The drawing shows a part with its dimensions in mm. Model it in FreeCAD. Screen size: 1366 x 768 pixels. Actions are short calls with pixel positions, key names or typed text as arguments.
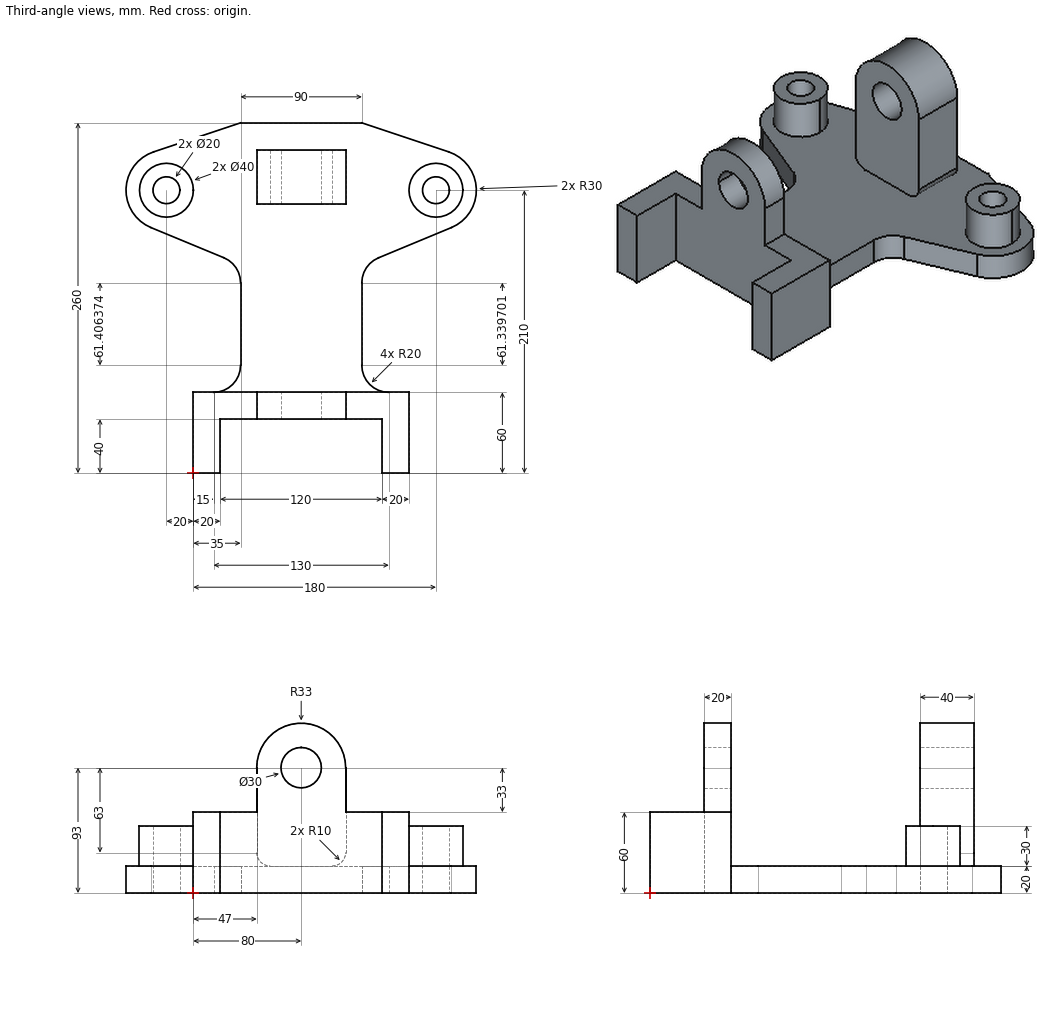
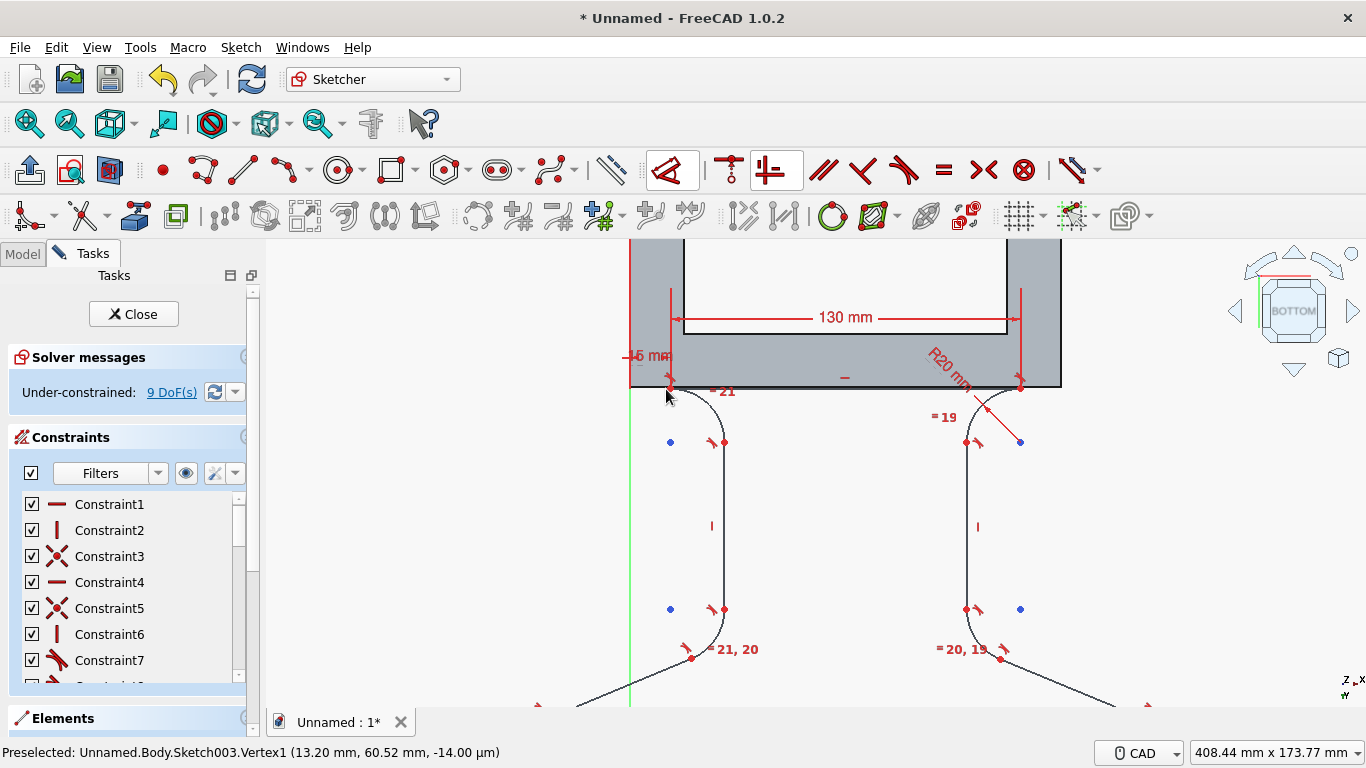
click(671, 389)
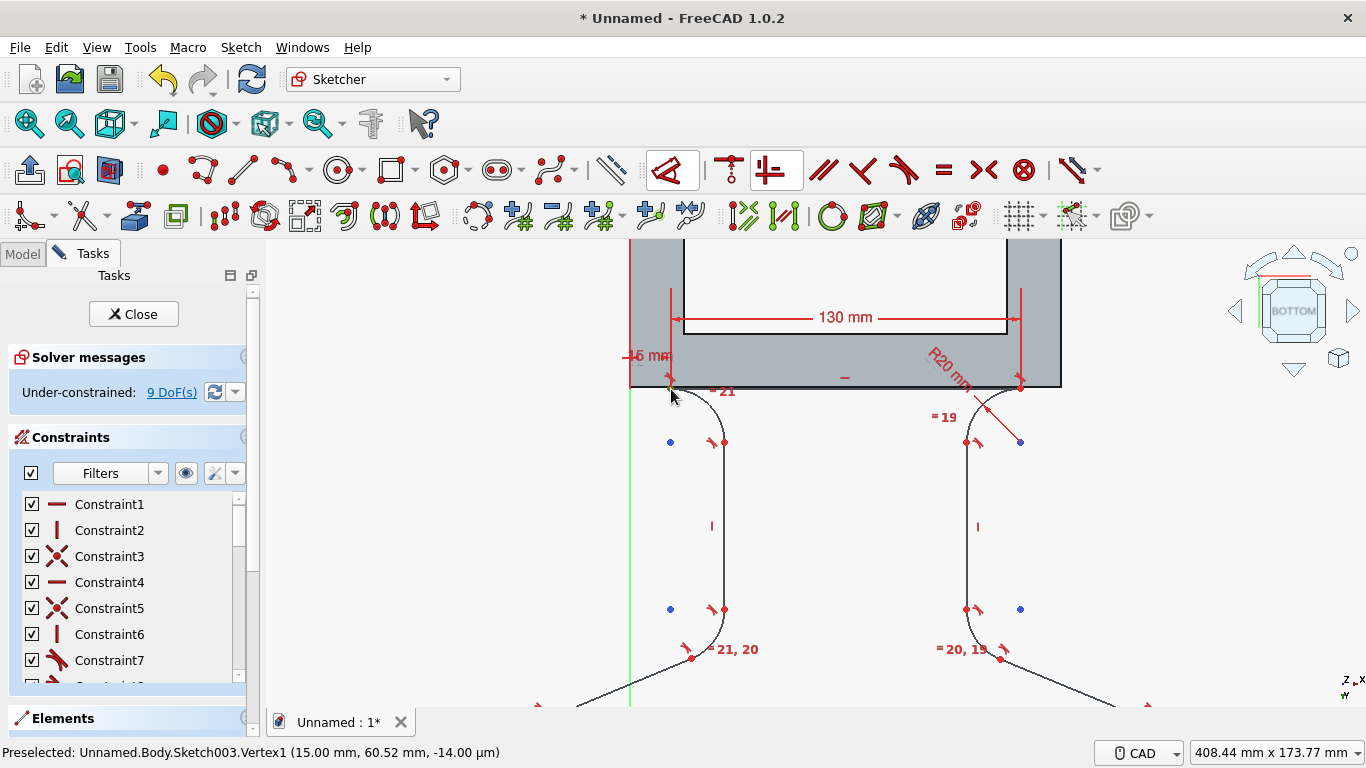
key(i)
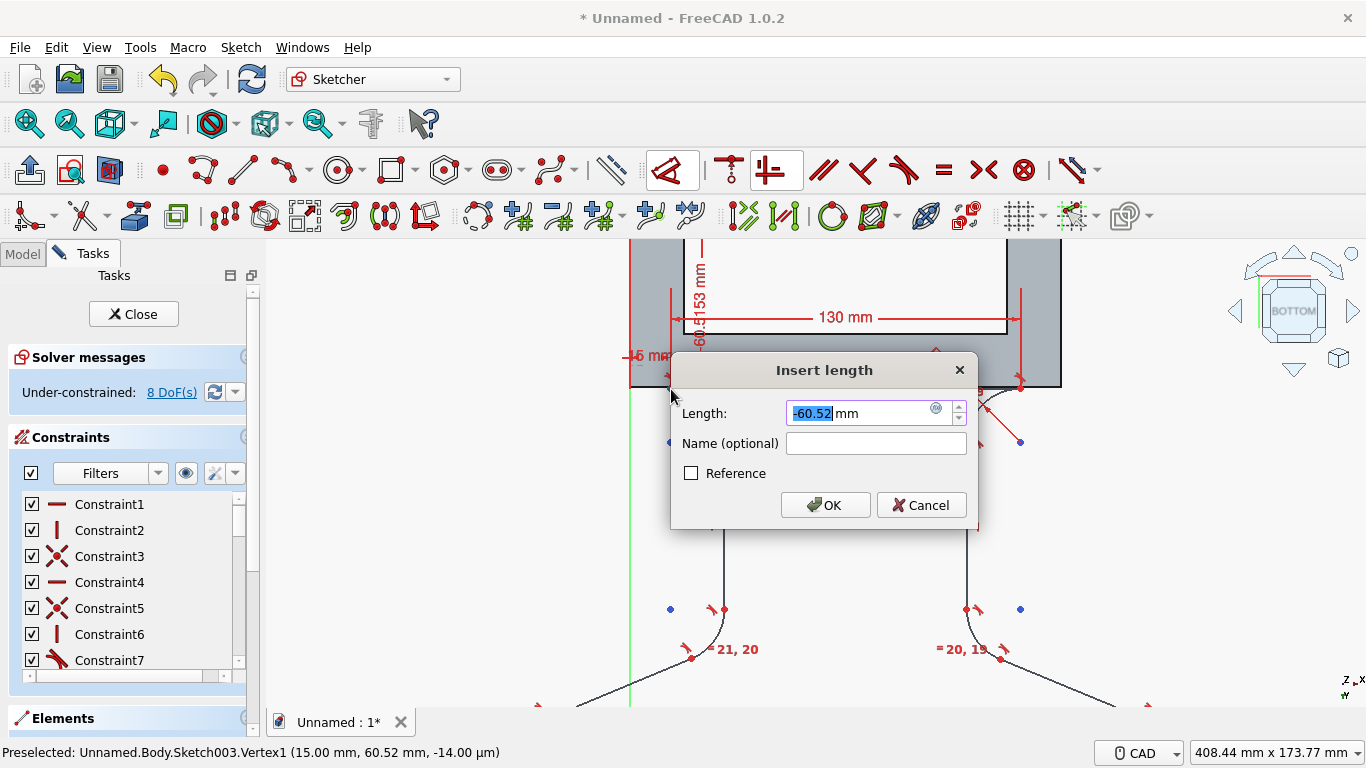
text(-60)
key(Return)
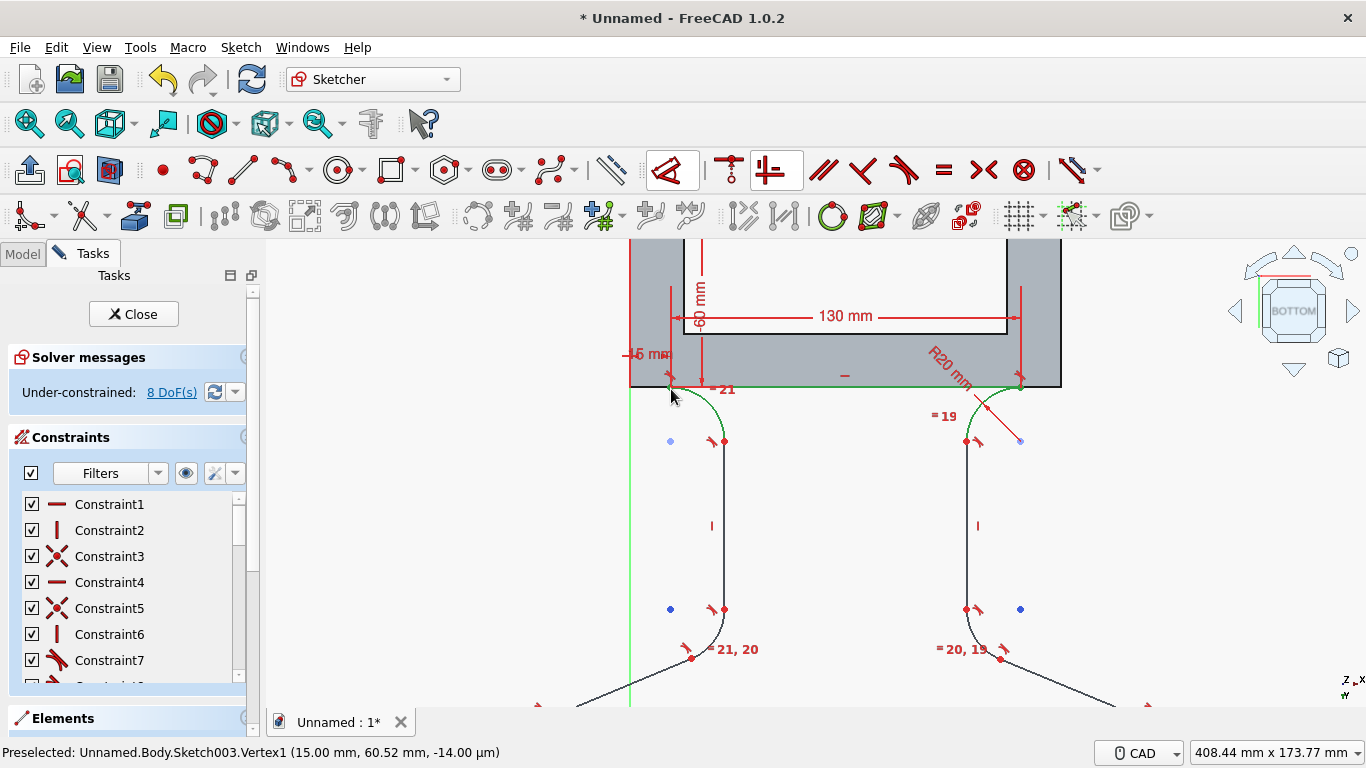
scroll(667, 389, down, 4)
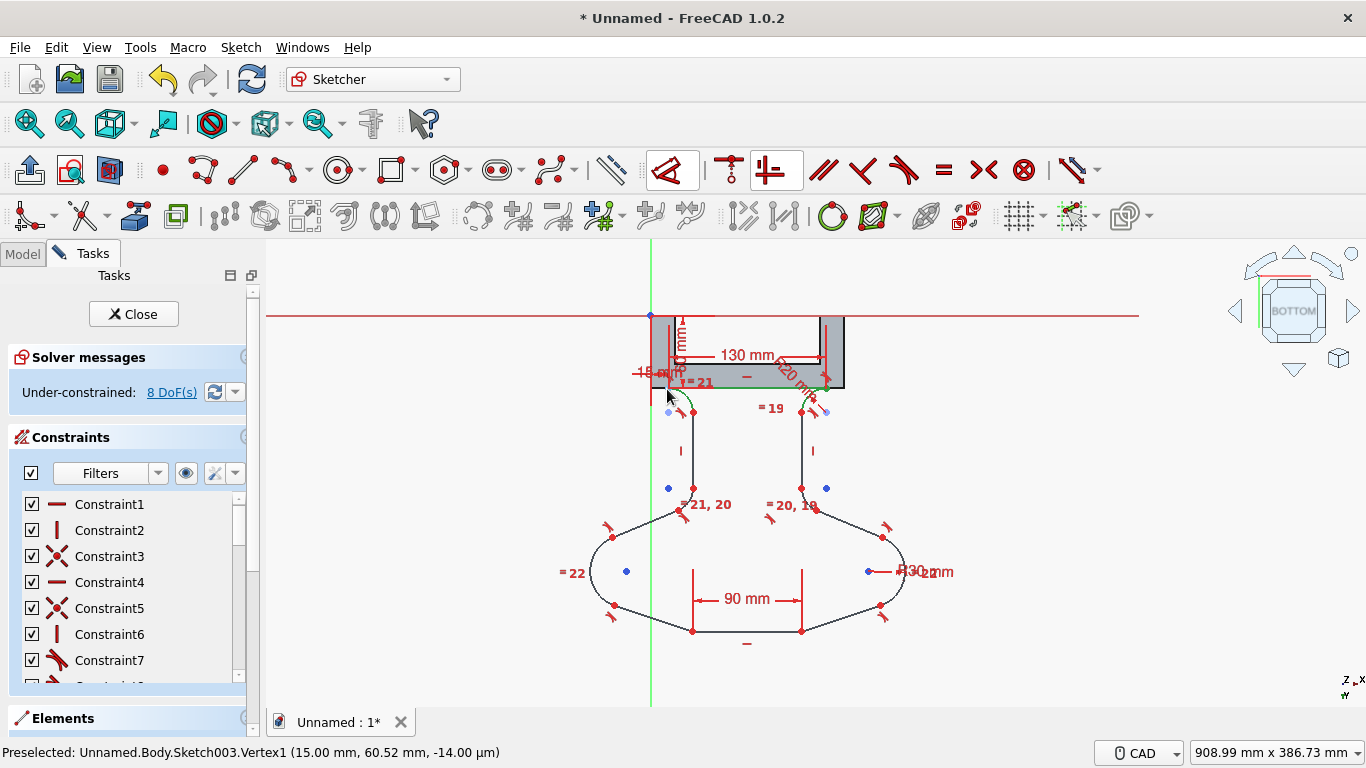
click(693, 632)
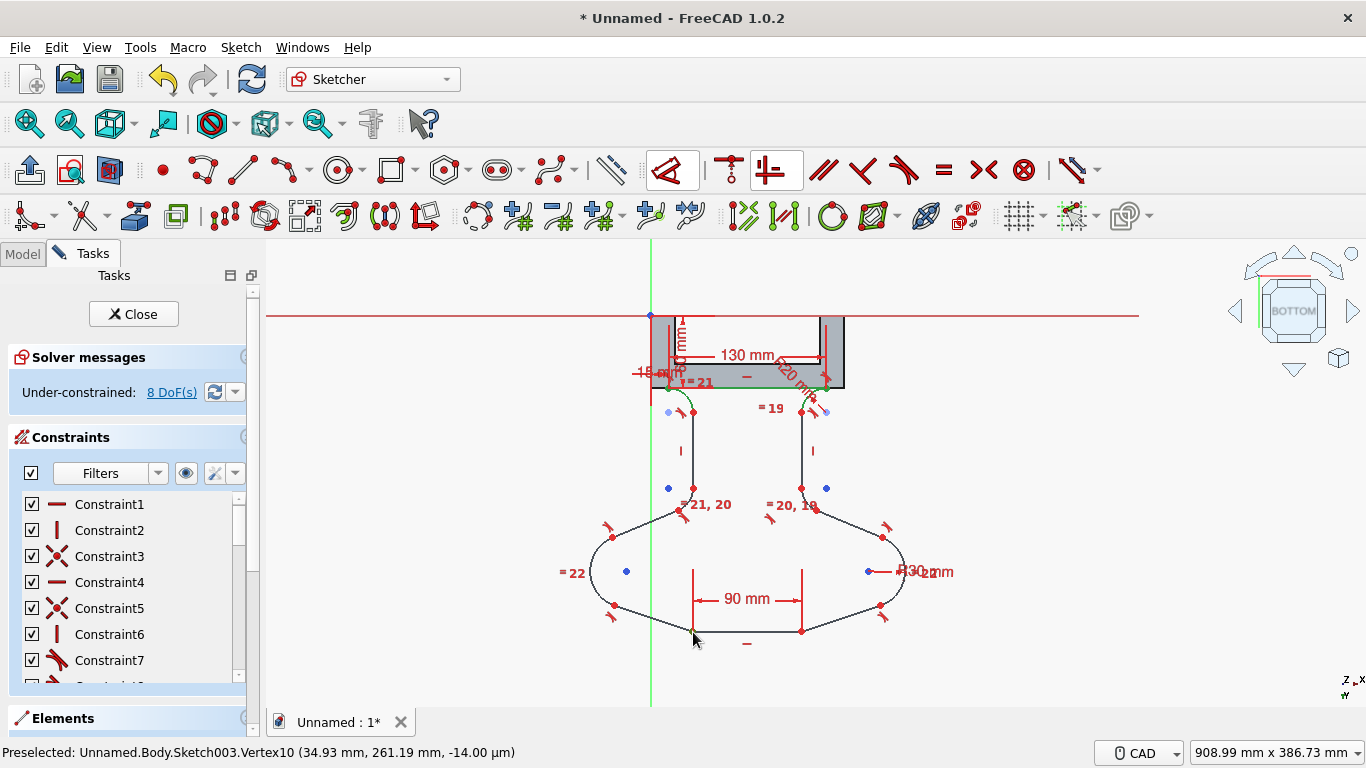
click(694, 170)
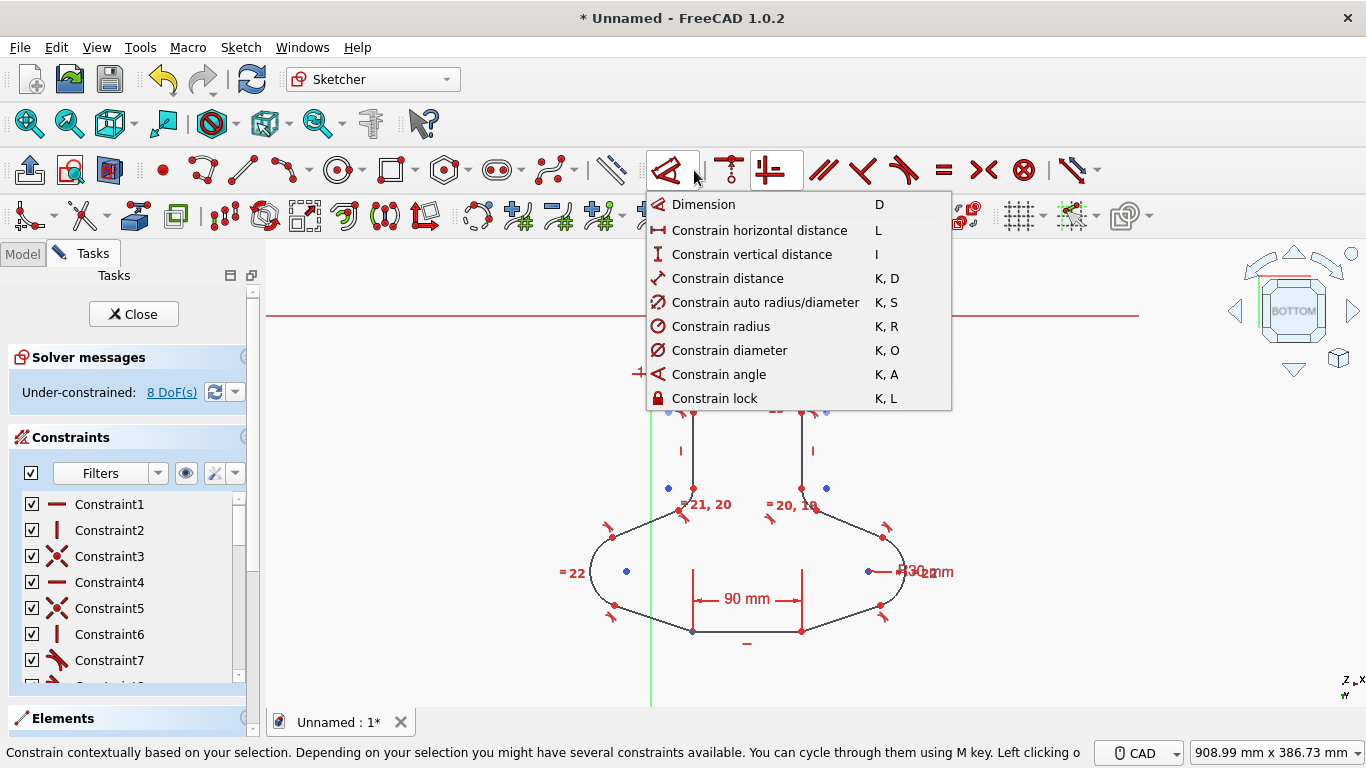
click(799, 230)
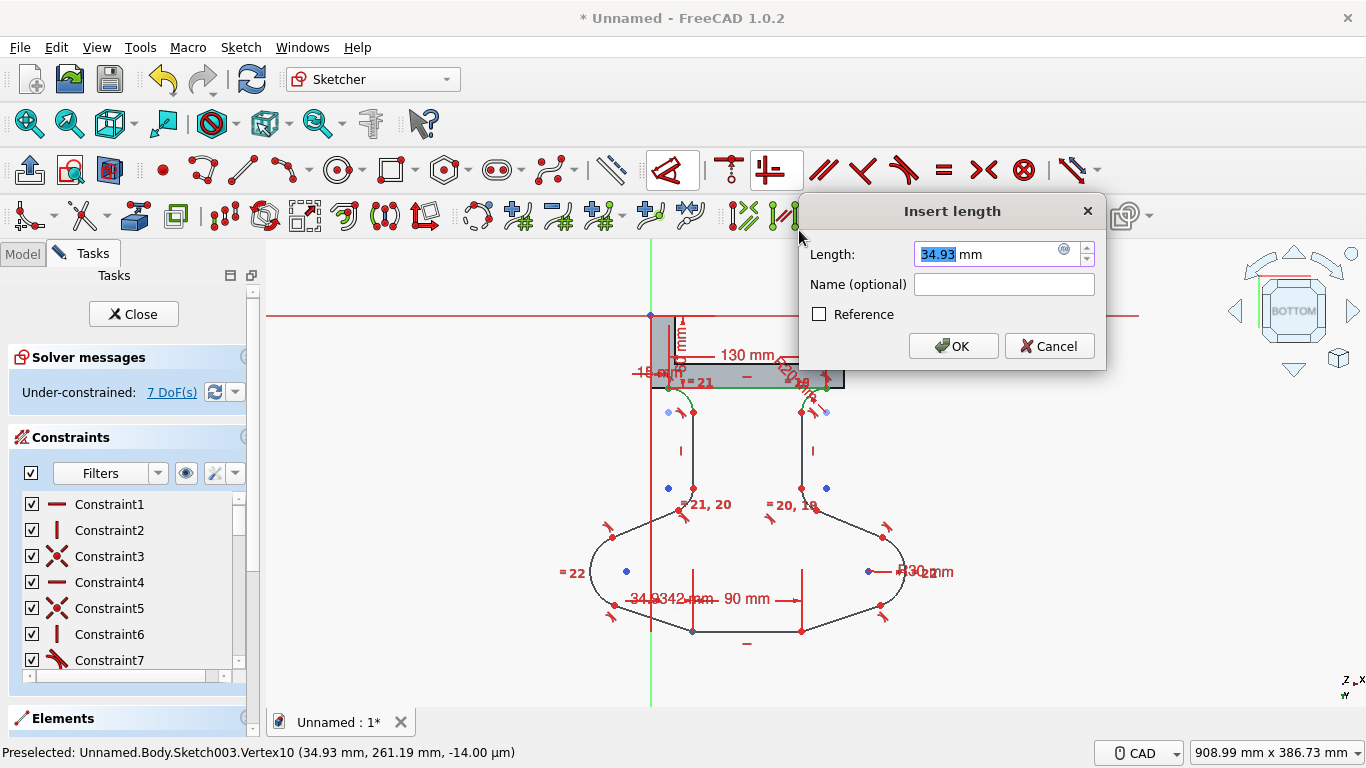
text(35)
key(Return)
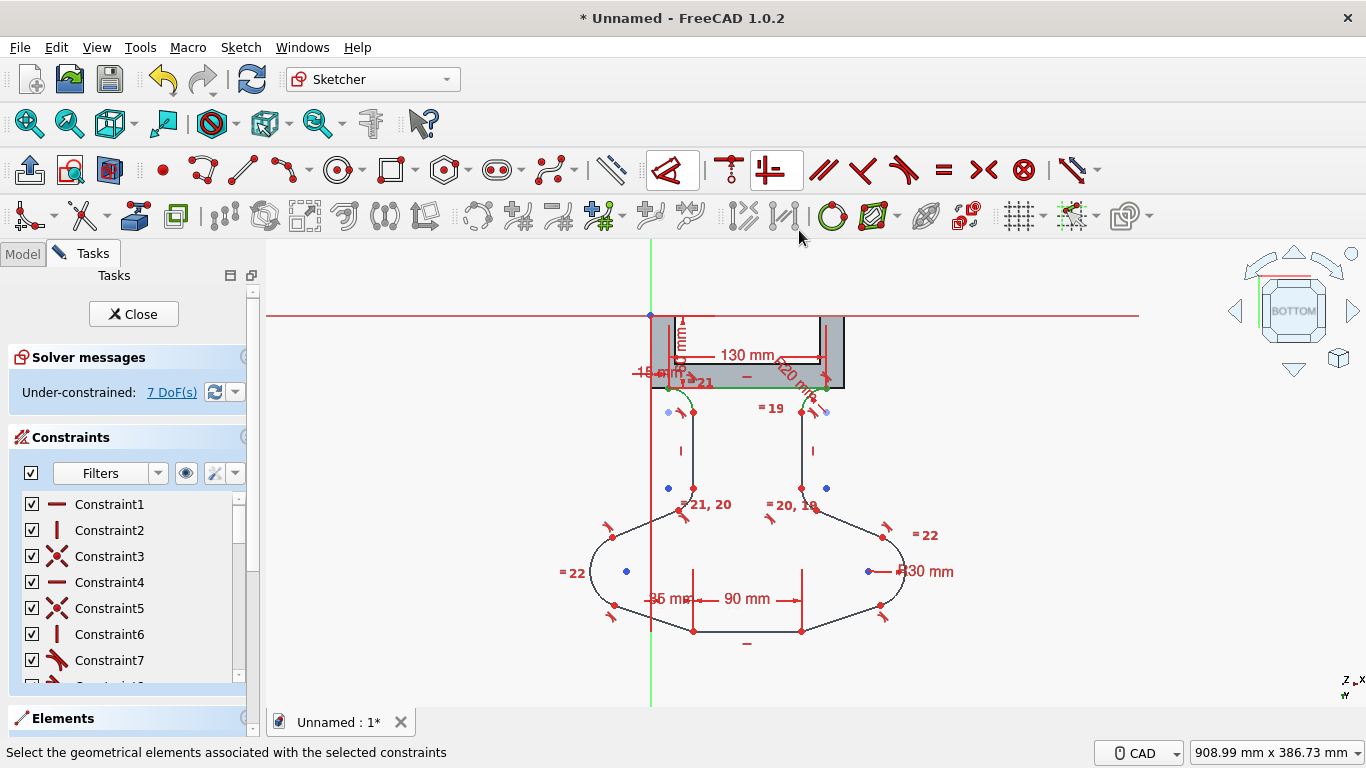
scroll(627, 571, up, 3)